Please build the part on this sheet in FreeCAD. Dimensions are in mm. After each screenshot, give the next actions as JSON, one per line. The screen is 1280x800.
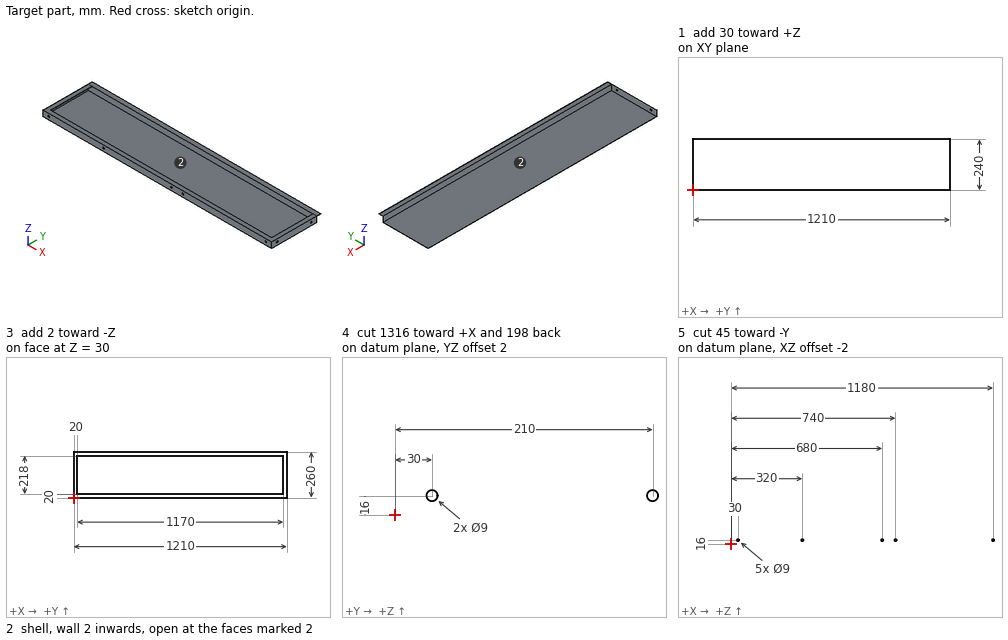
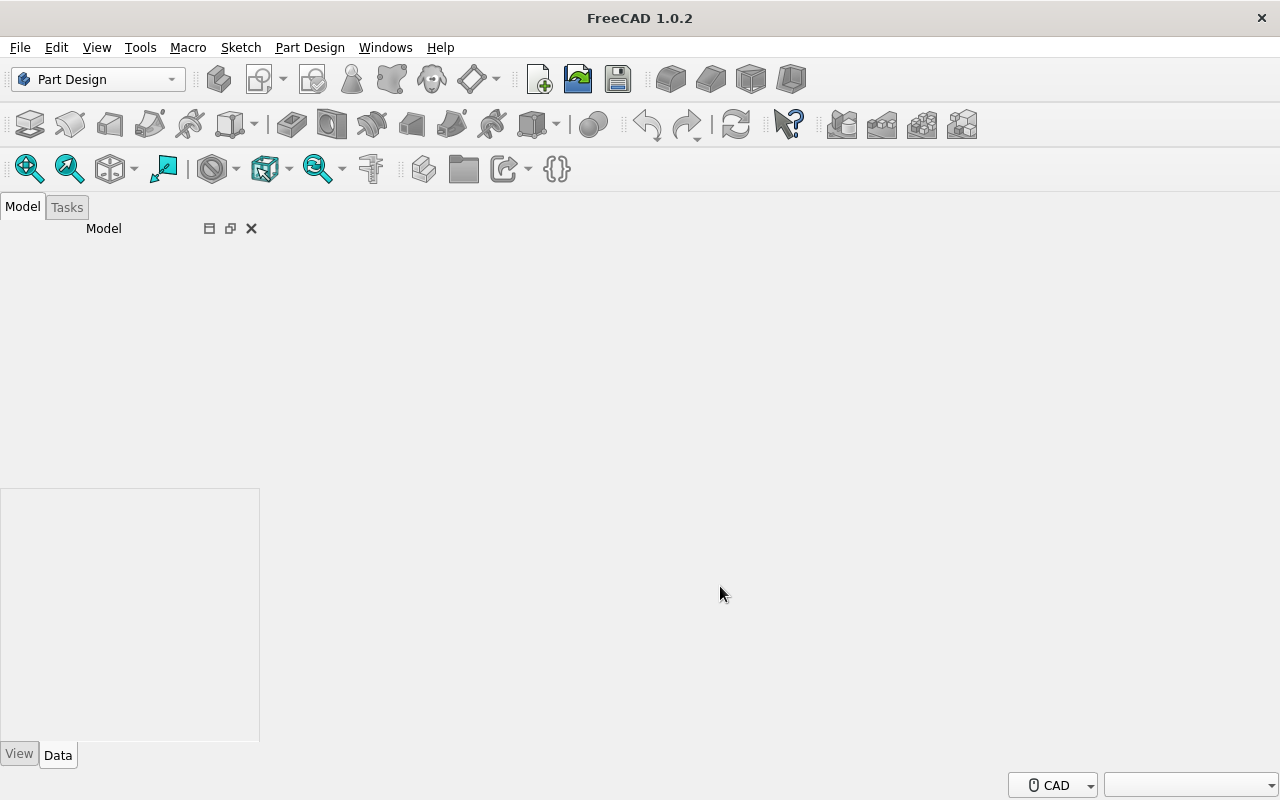
{"action": "key", "text": "ctrl+n"}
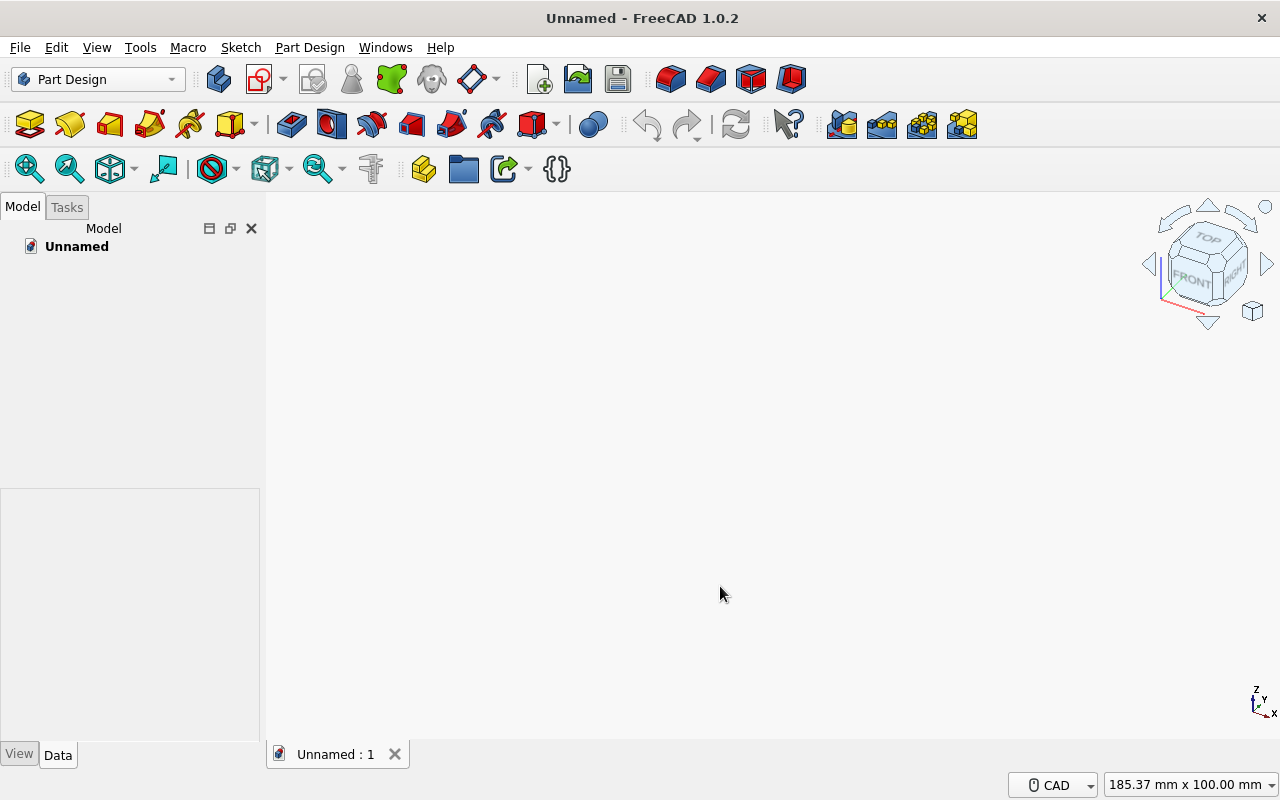
{"action": "left_click", "coordinate": [260, 80]}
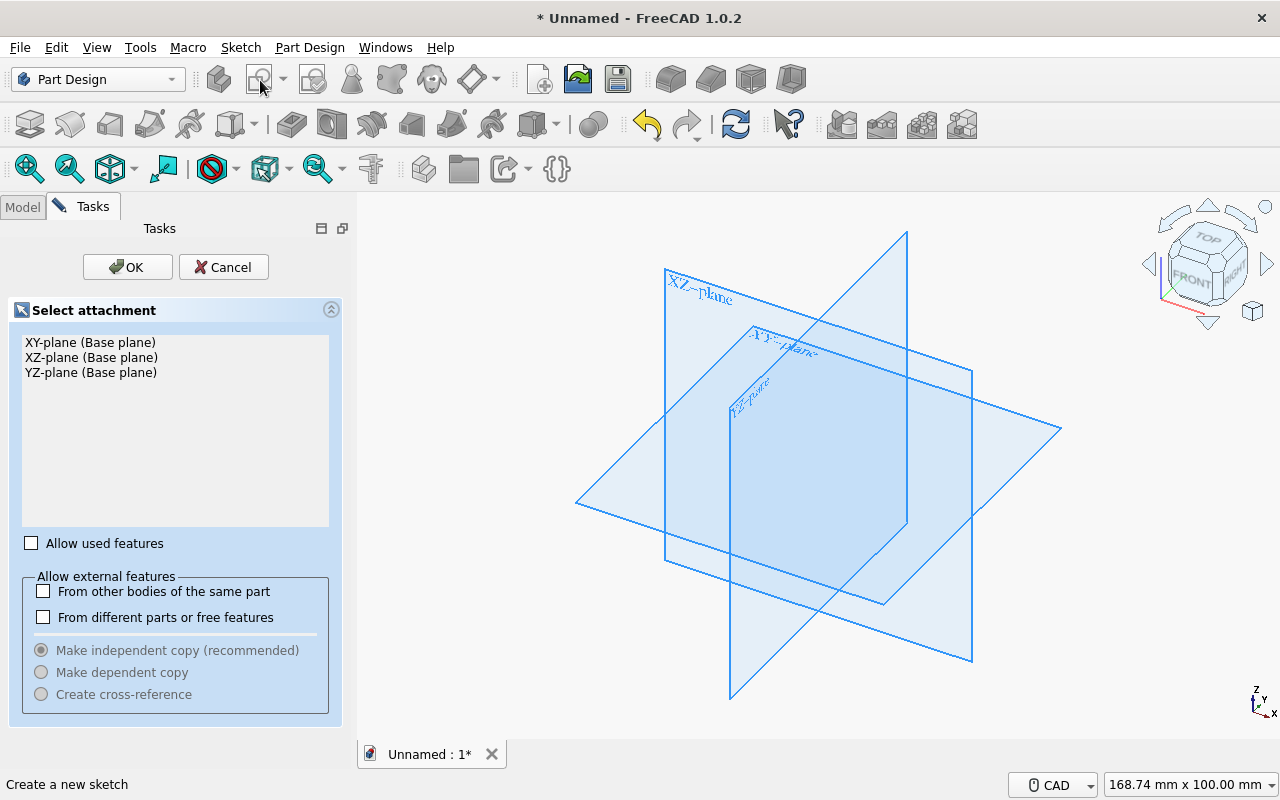
{"action": "left_click", "coordinate": [82, 342]}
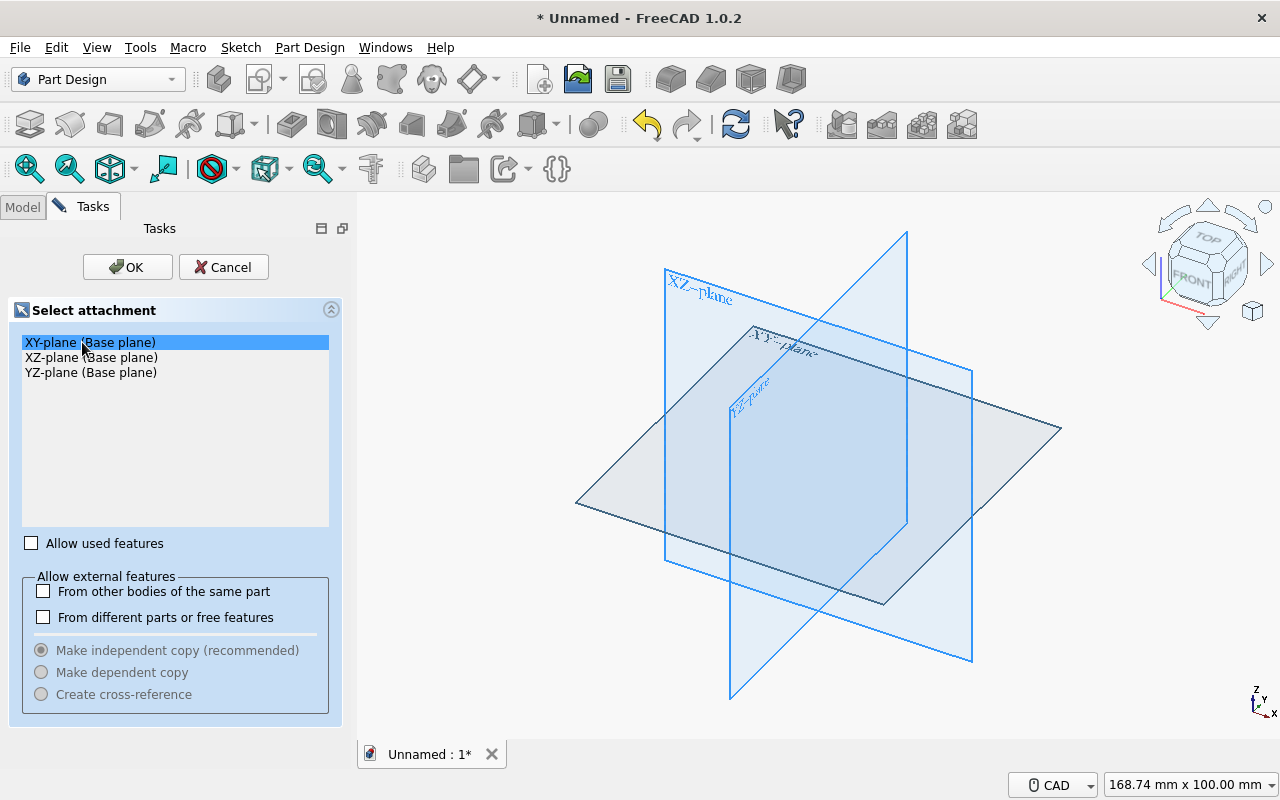
{"action": "left_click", "coordinate": [128, 267]}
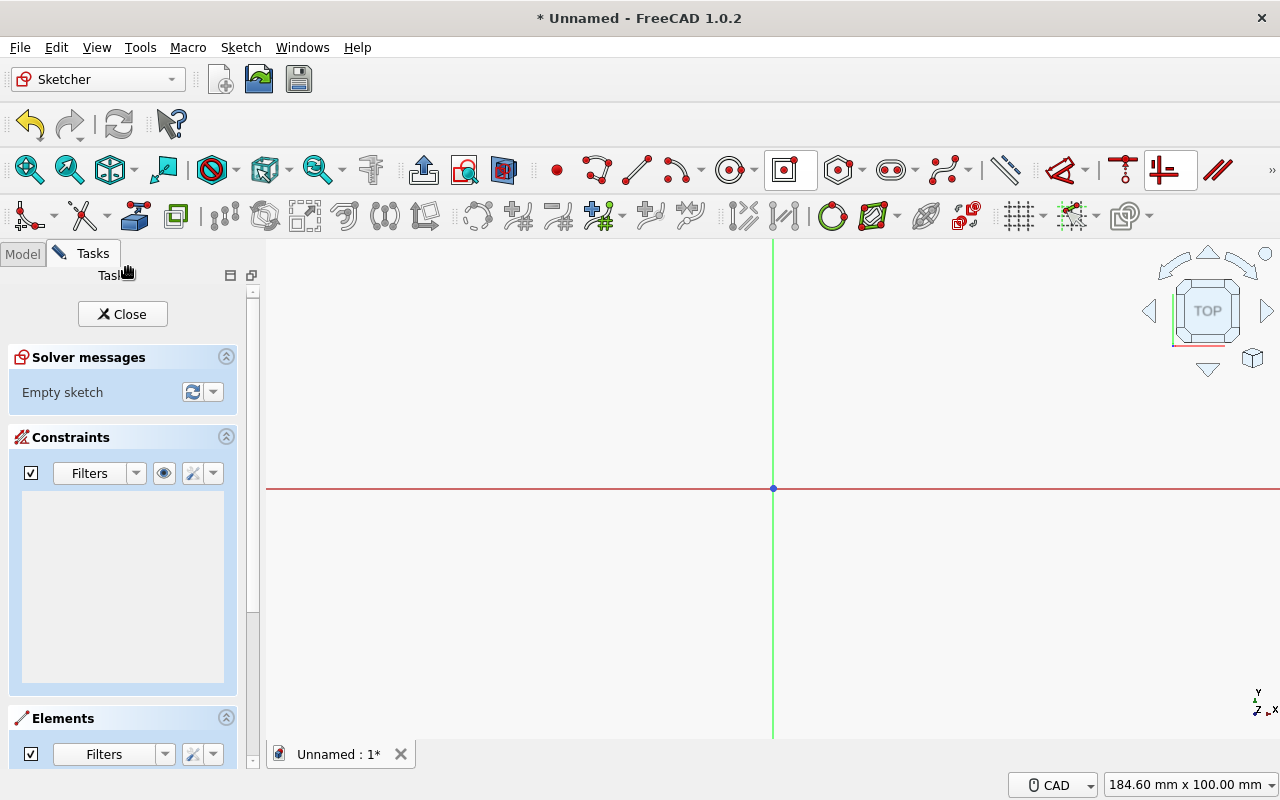
{"action": "scroll", "coordinate": [396, 549], "scroll_direction": "down", "scroll_amount": 12}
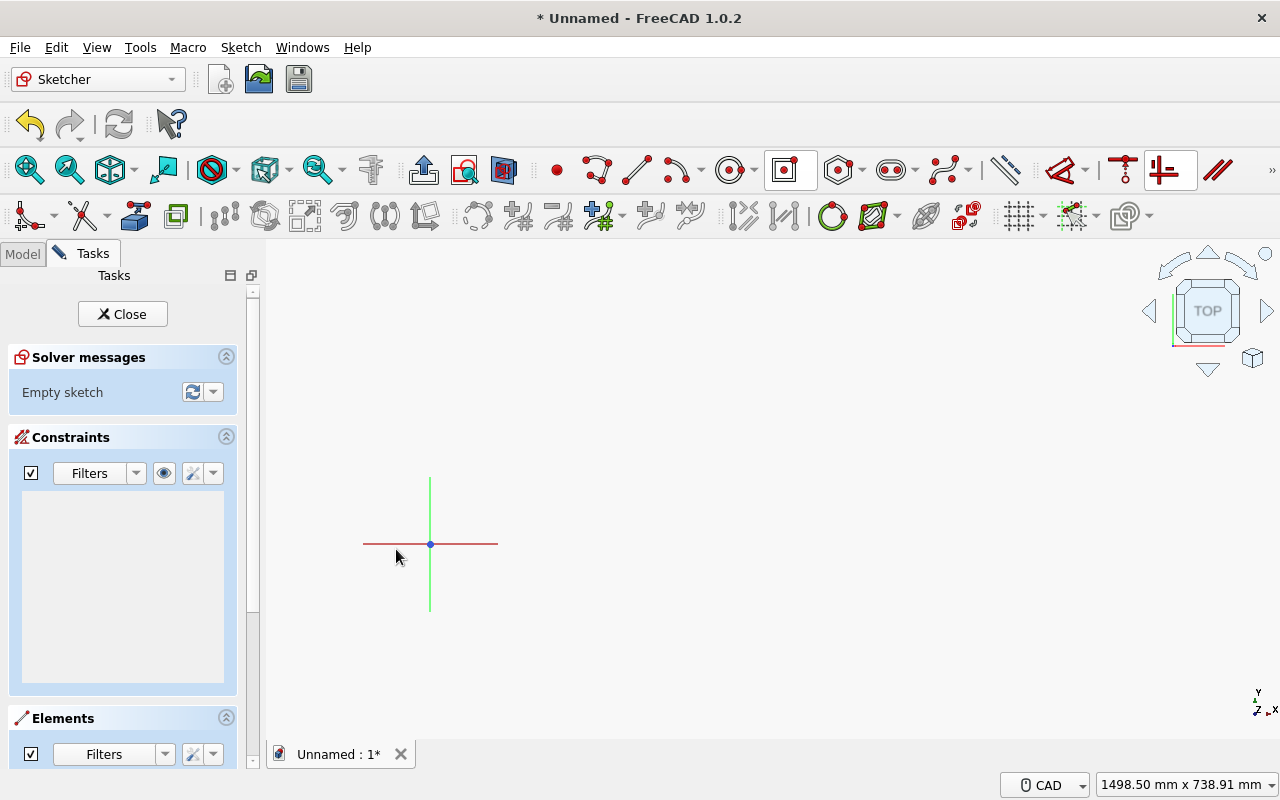
{"action": "key", "text": "g r"}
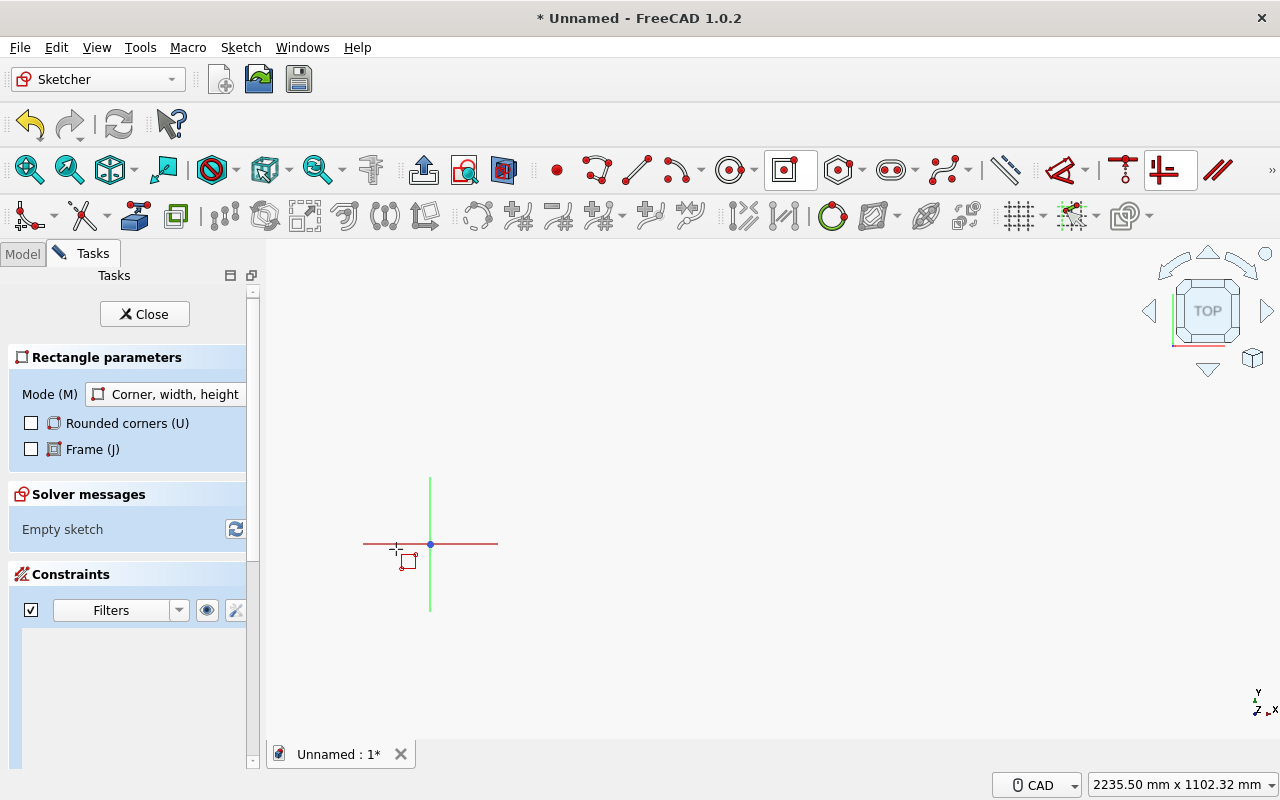
{"action": "left_click", "coordinate": [430, 544]}
{"action": "mouse_move", "coordinate": [979, 435]}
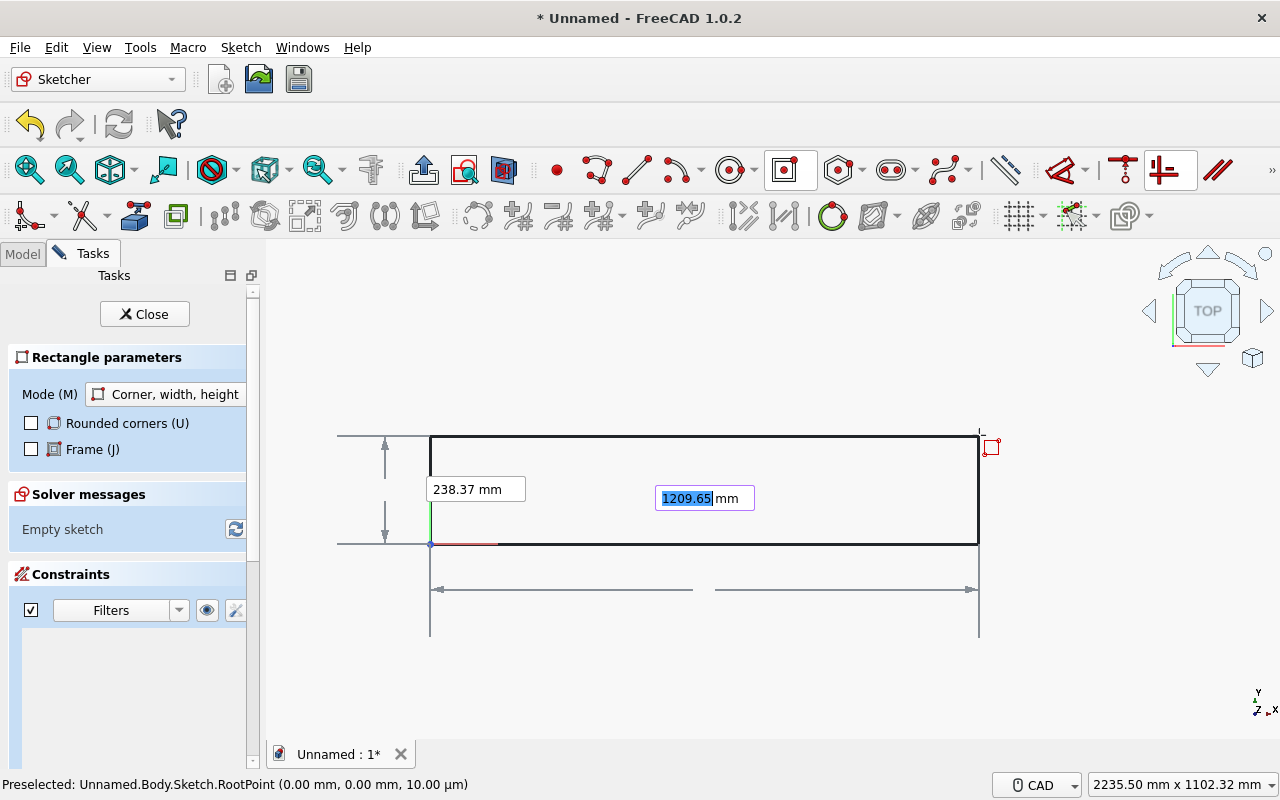
{"action": "type", "text": "1210"}
{"action": "key", "text": "Tab"}
{"action": "type", "text": "240"}
{"action": "key", "text": "Return"}
{"action": "key", "text": "Escape"}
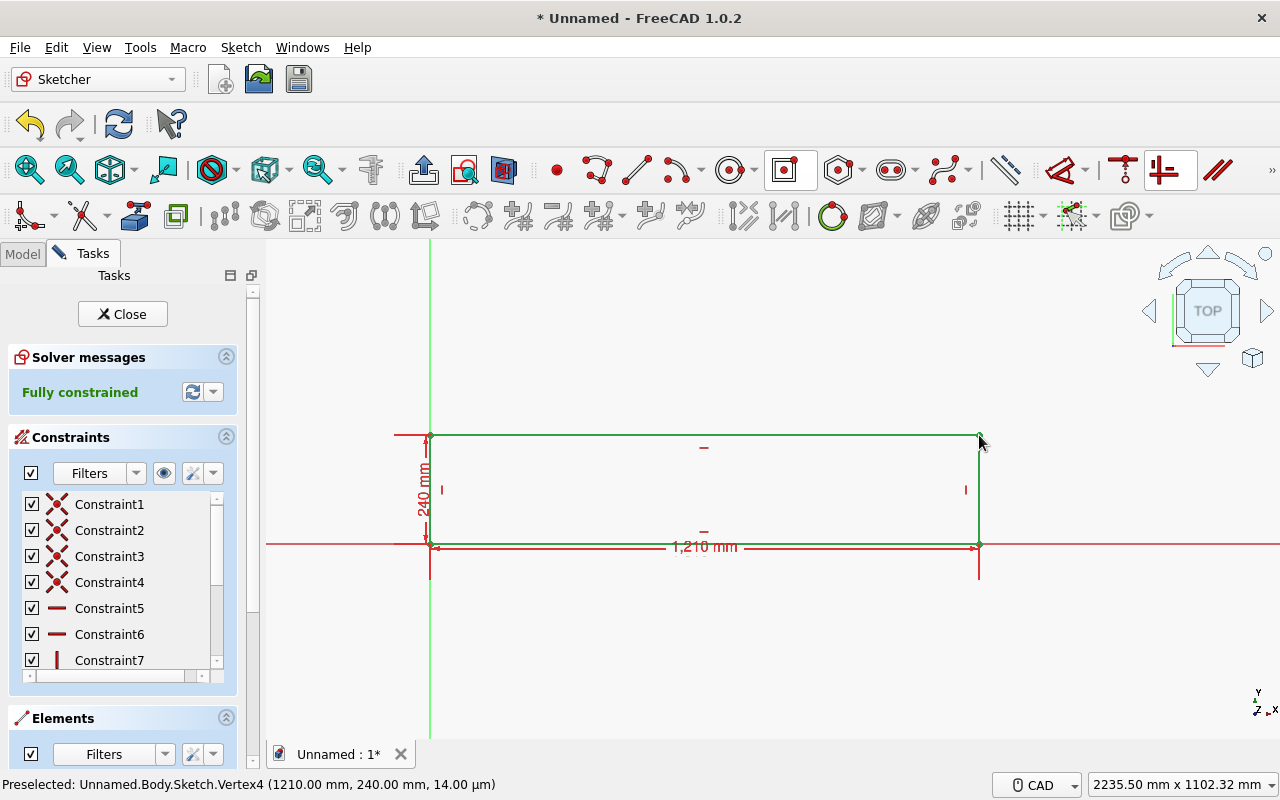
{"action": "left_click", "coordinate": [123, 314]}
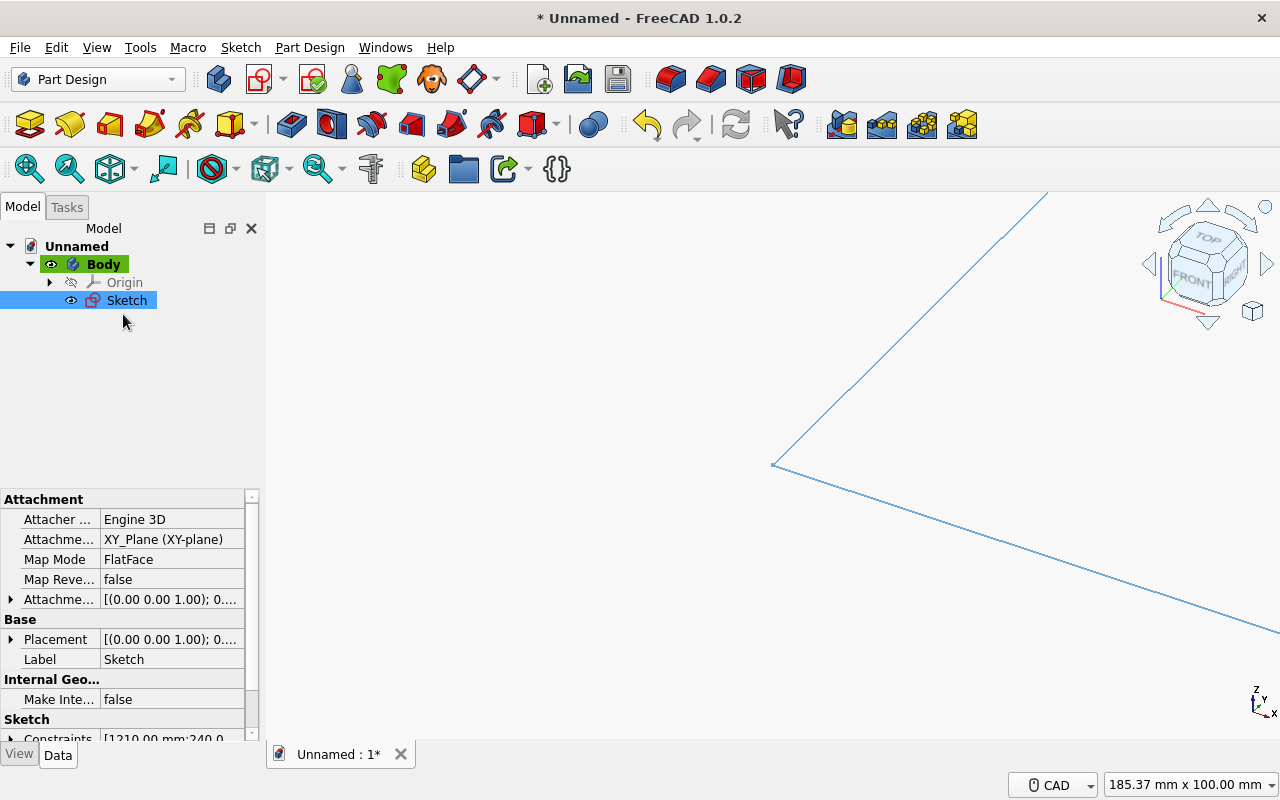
{"action": "left_click", "coordinate": [30, 124]}